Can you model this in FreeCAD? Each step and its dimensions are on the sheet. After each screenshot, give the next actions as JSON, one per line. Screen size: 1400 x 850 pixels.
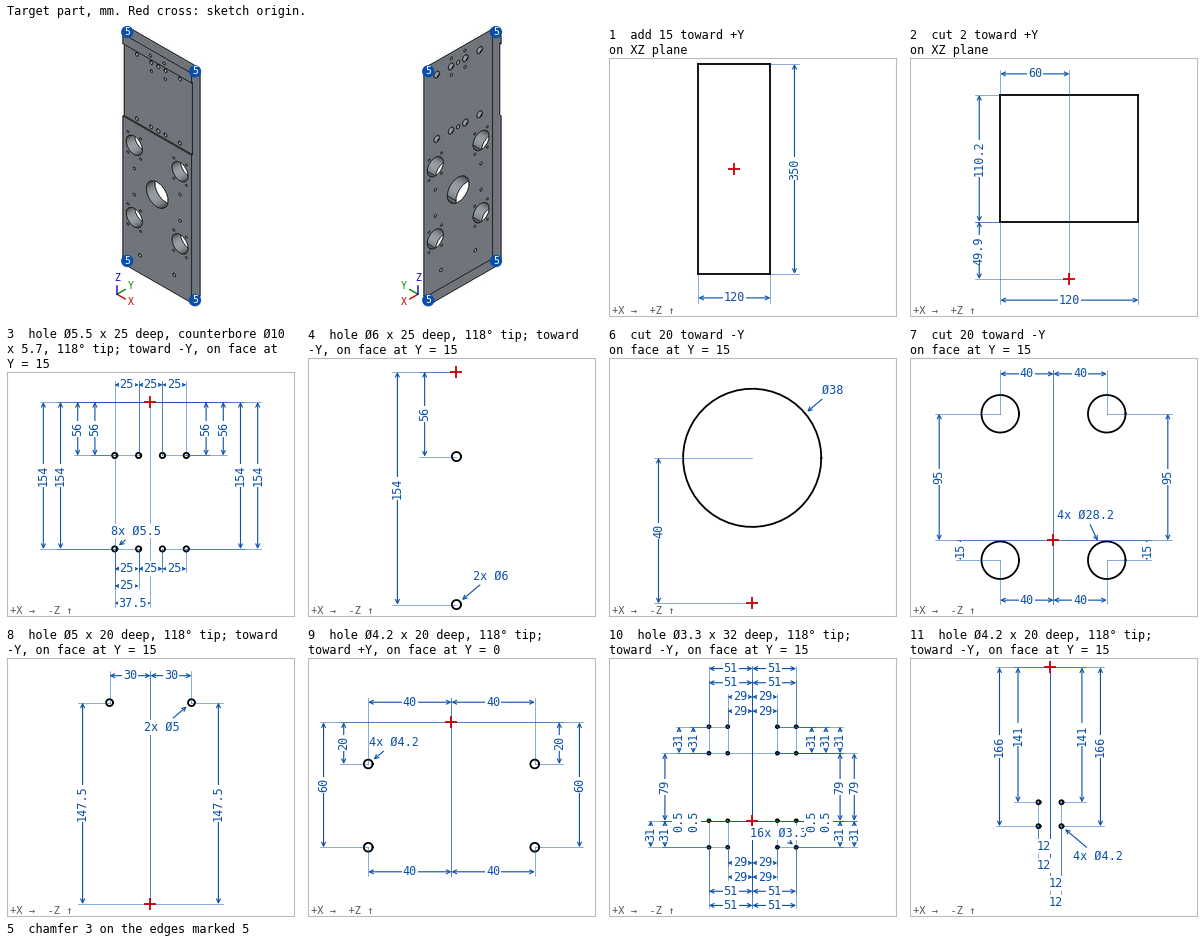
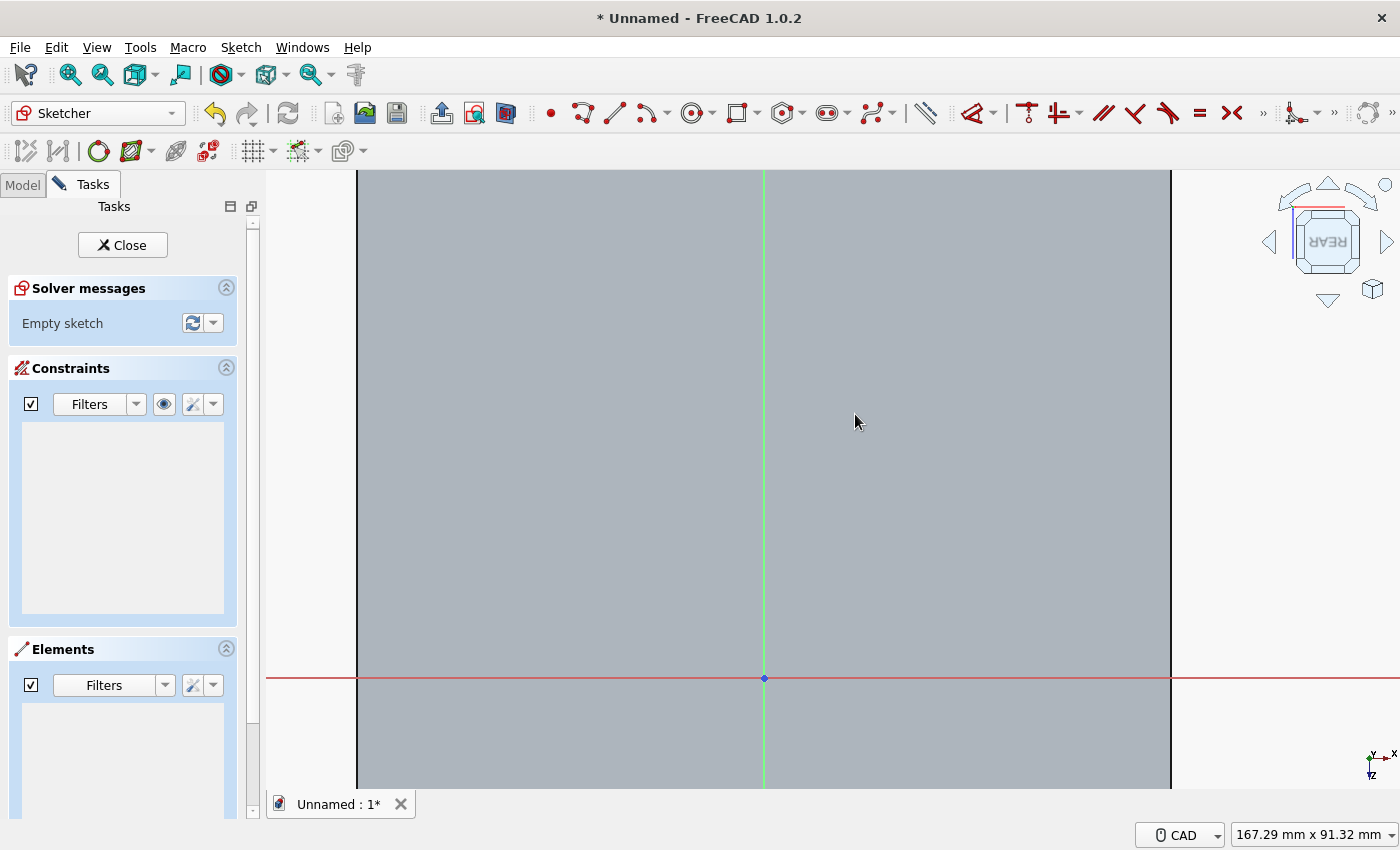
{"action": "left_click", "coordinate": [692, 114]}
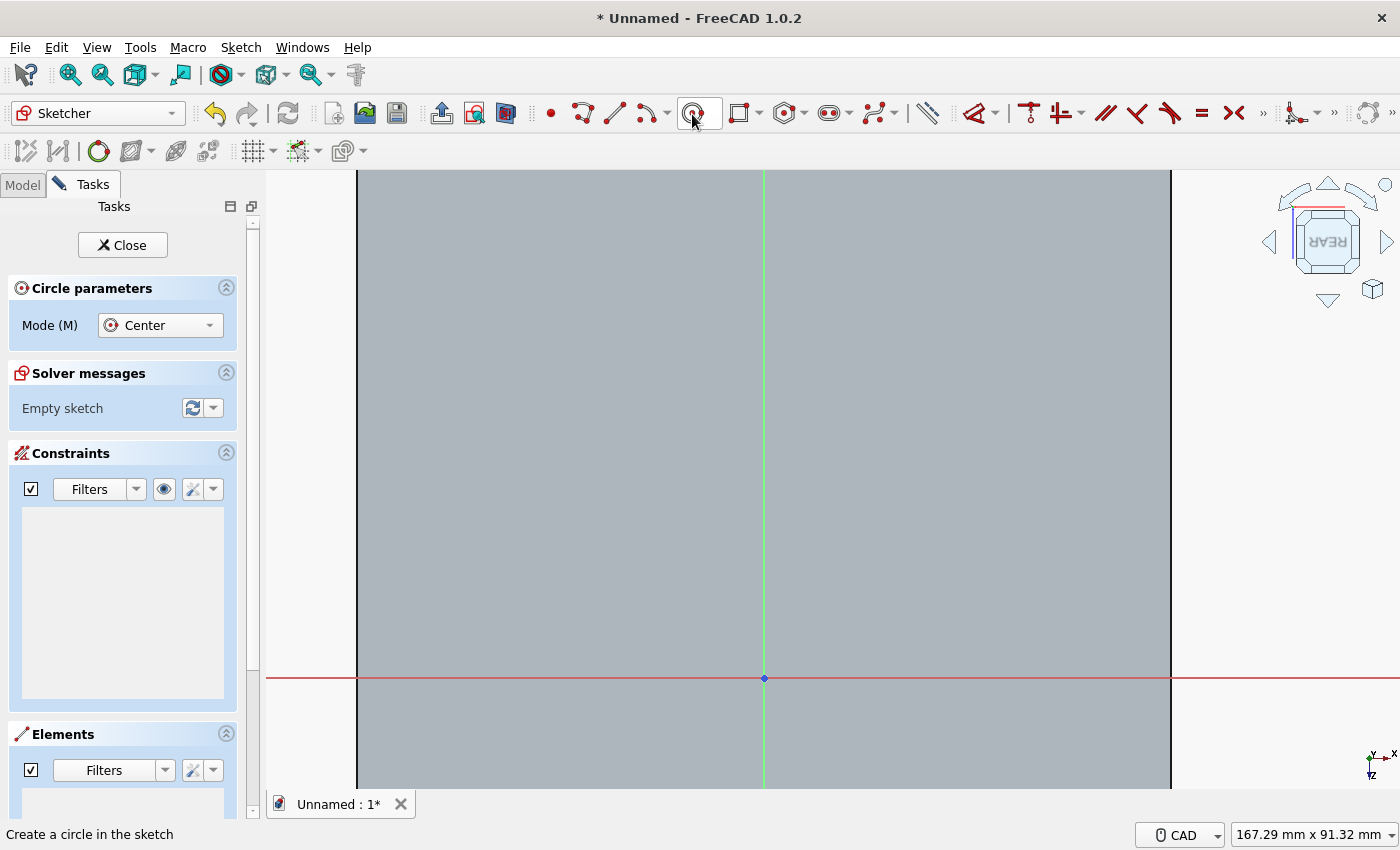
{"action": "left_click", "coordinate": [764, 407]}
{"action": "left_click", "coordinate": [855, 316]}
{"action": "key", "text": "Escape"}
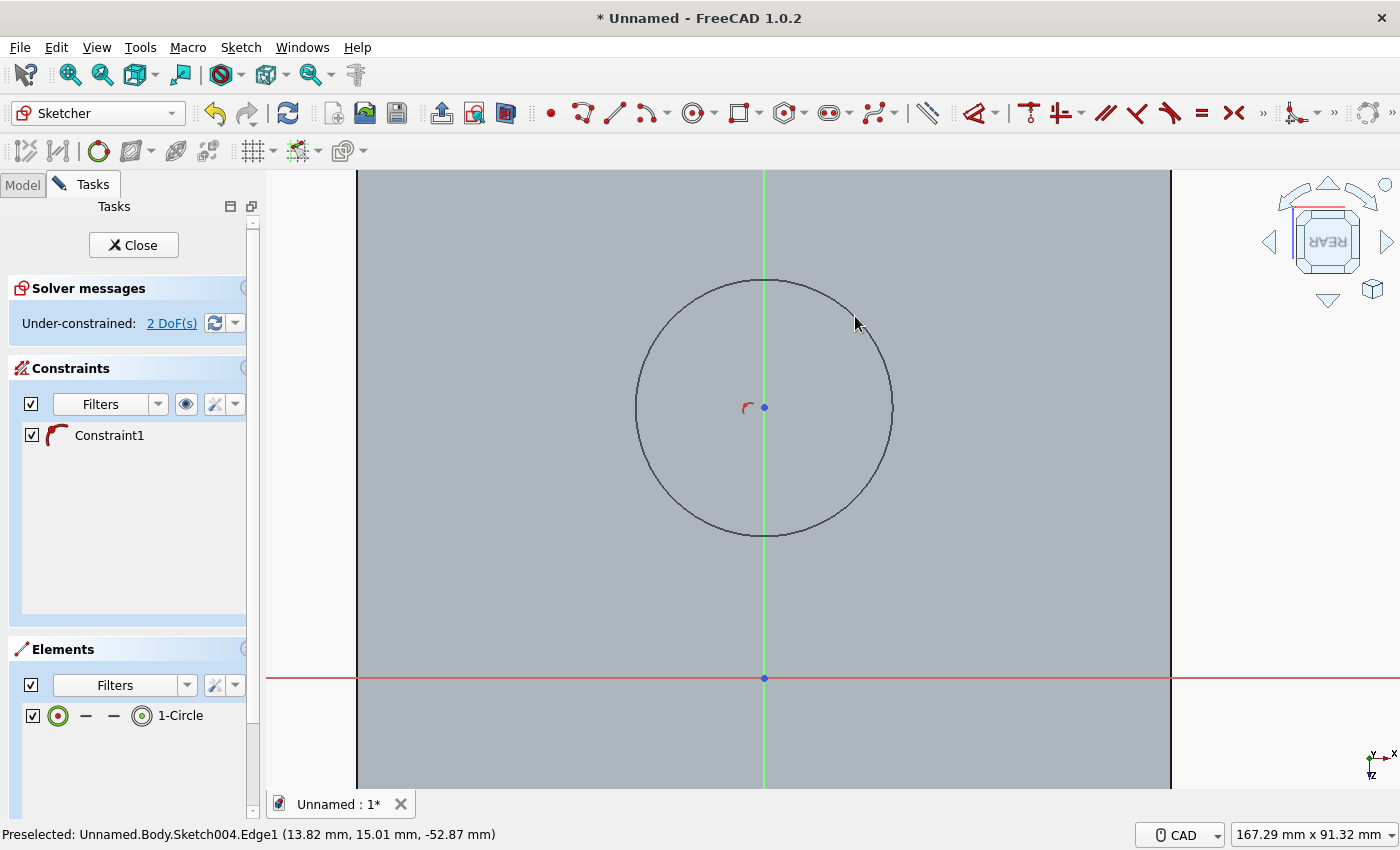
{"action": "left_click", "coordinate": [974, 114]}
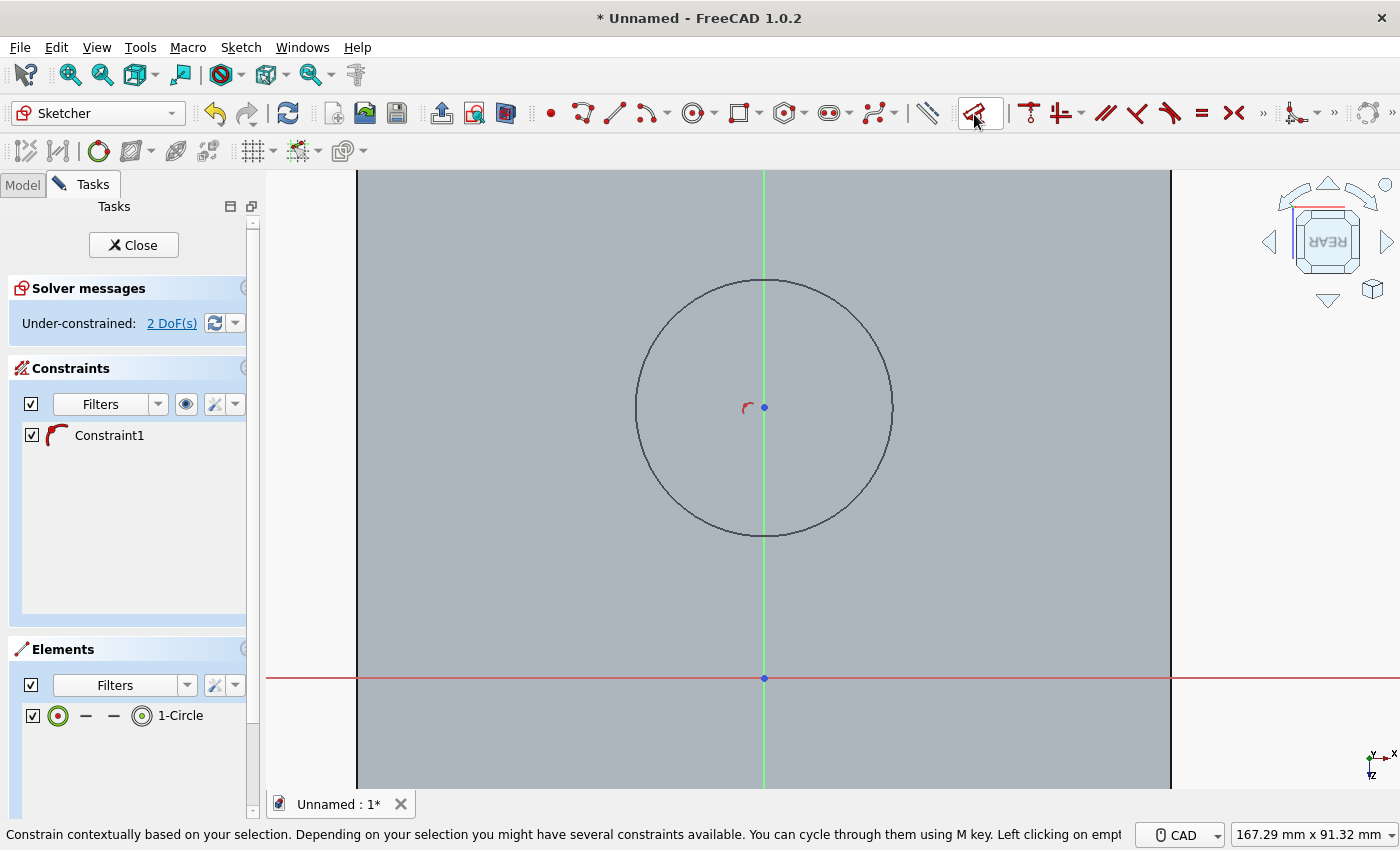
{"action": "left_click", "coordinate": [855, 317]}
{"action": "left_click", "coordinate": [878, 294]}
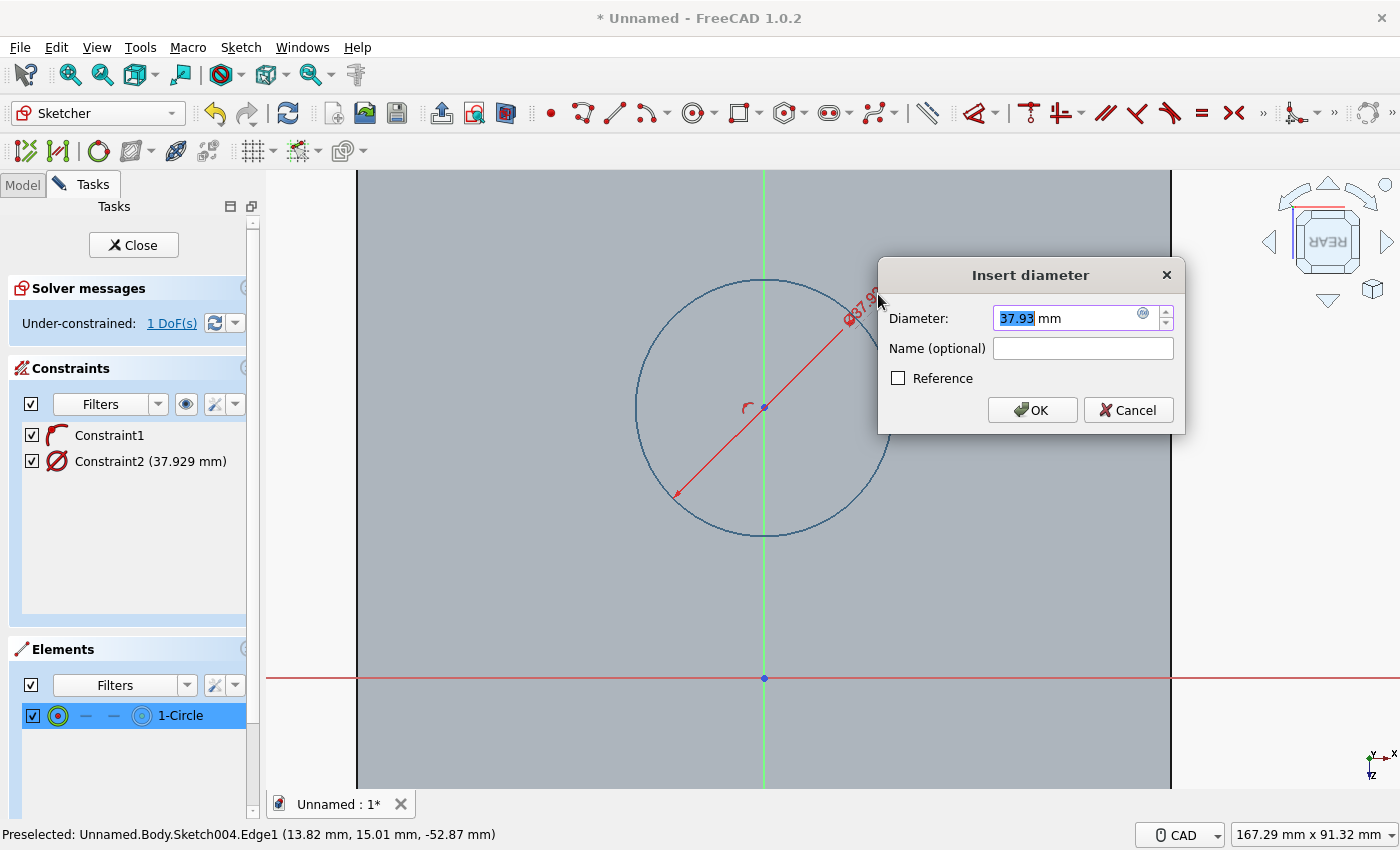
{"action": "type", "text": "38"}
{"action": "key", "text": "Return"}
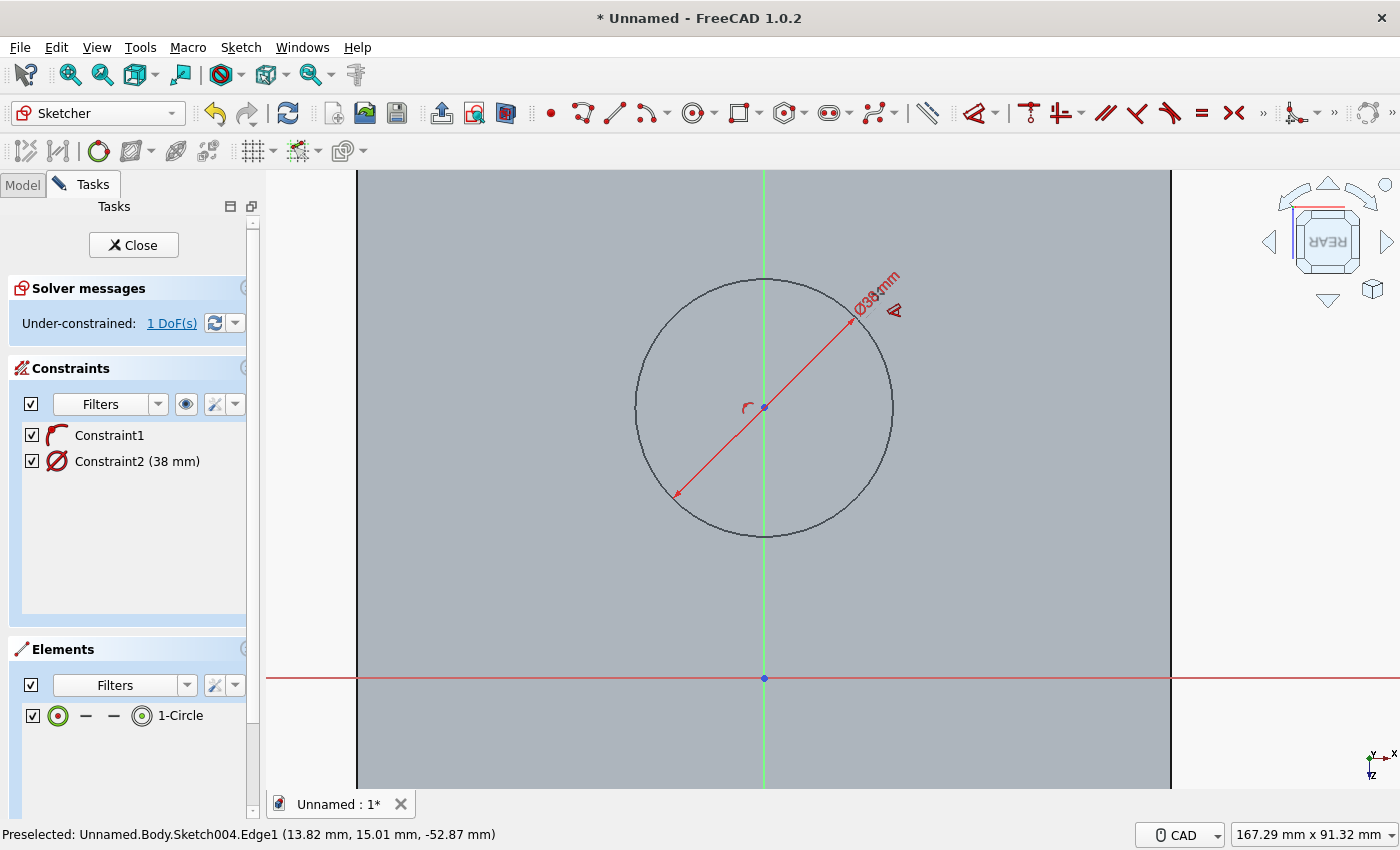
{"action": "left_click", "coordinate": [764, 408]}
{"action": "left_click", "coordinate": [798, 481]}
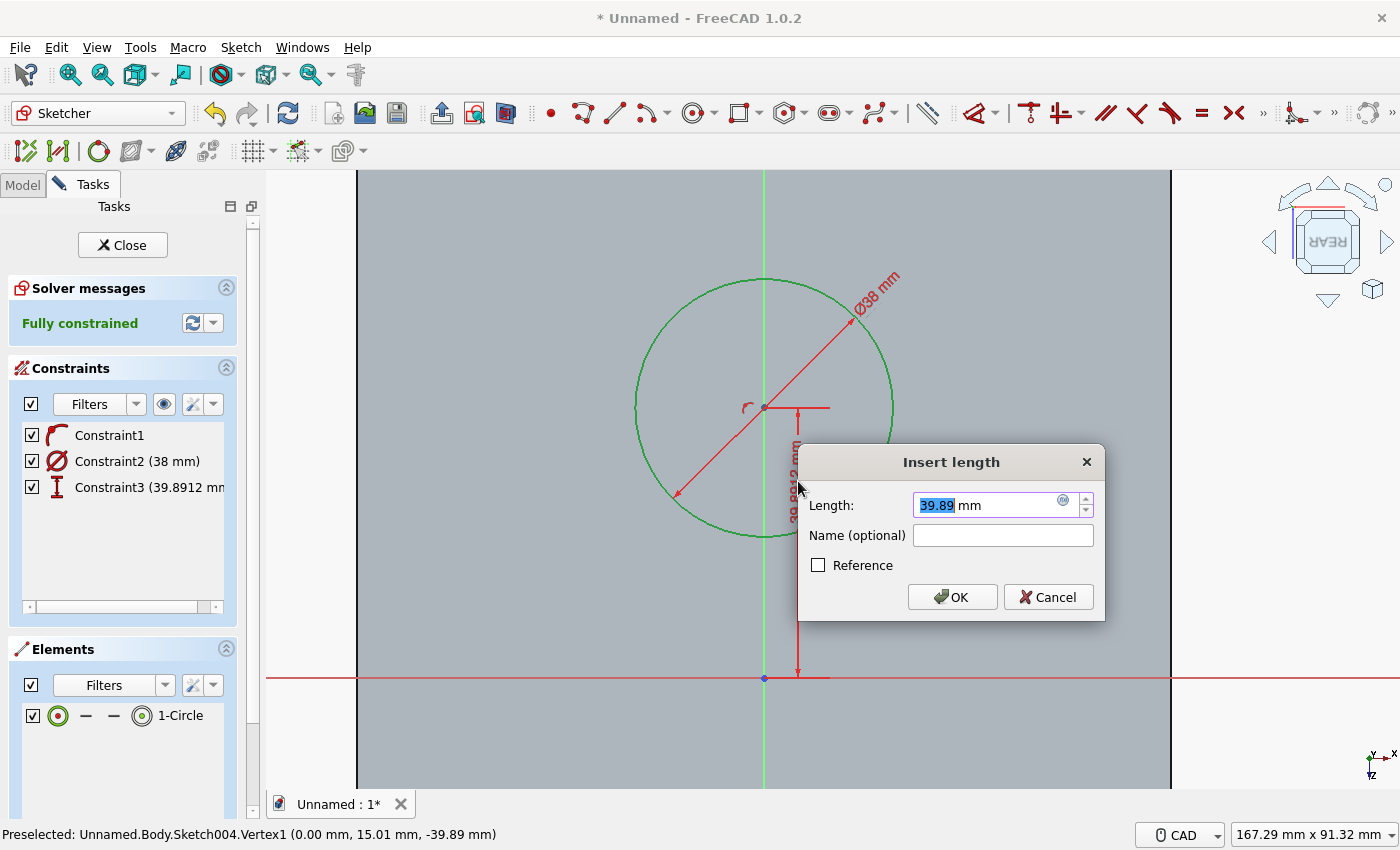
{"action": "type", "text": "40"}
{"action": "key", "text": "Return"}
{"action": "key", "text": "Escape"}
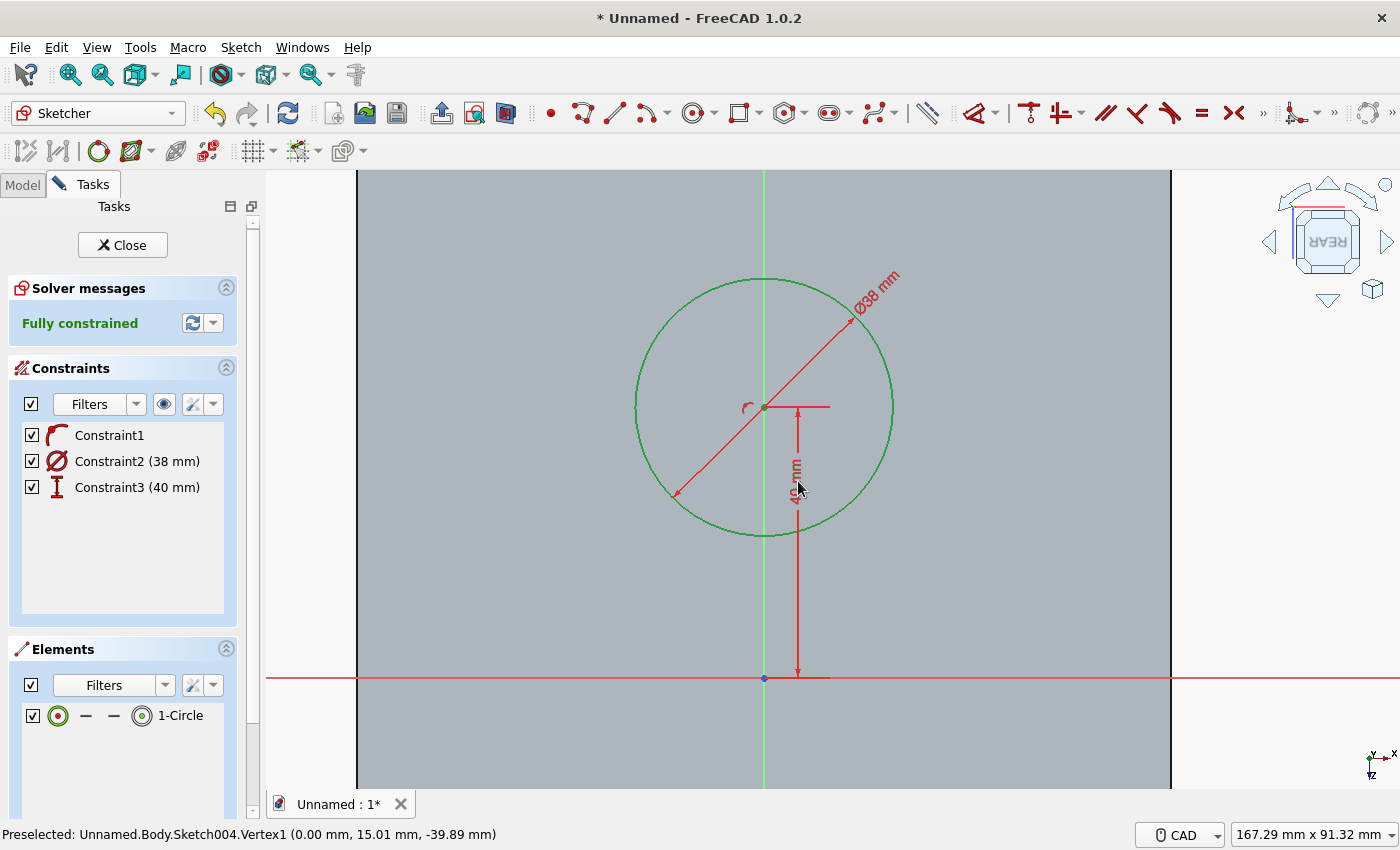
{"action": "left_click", "coordinate": [123, 245]}